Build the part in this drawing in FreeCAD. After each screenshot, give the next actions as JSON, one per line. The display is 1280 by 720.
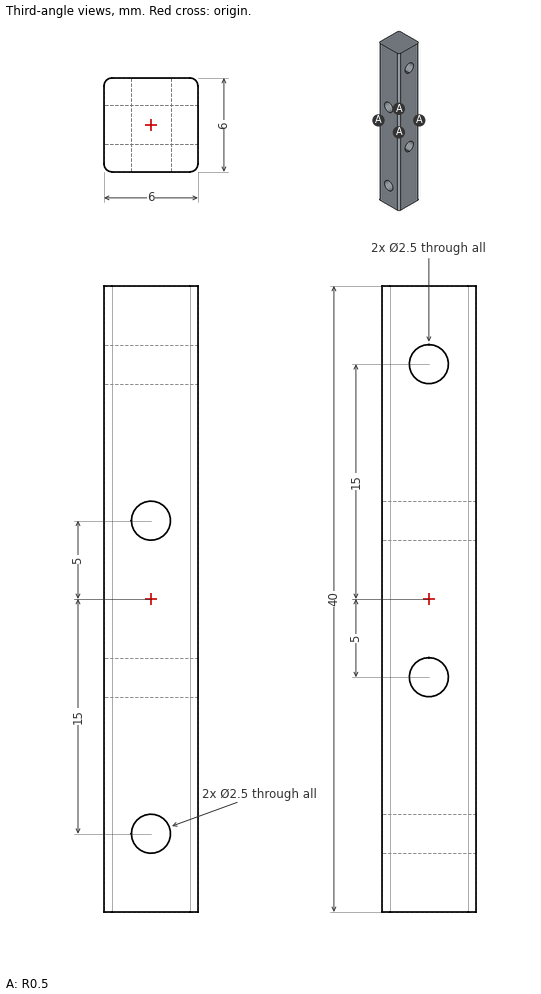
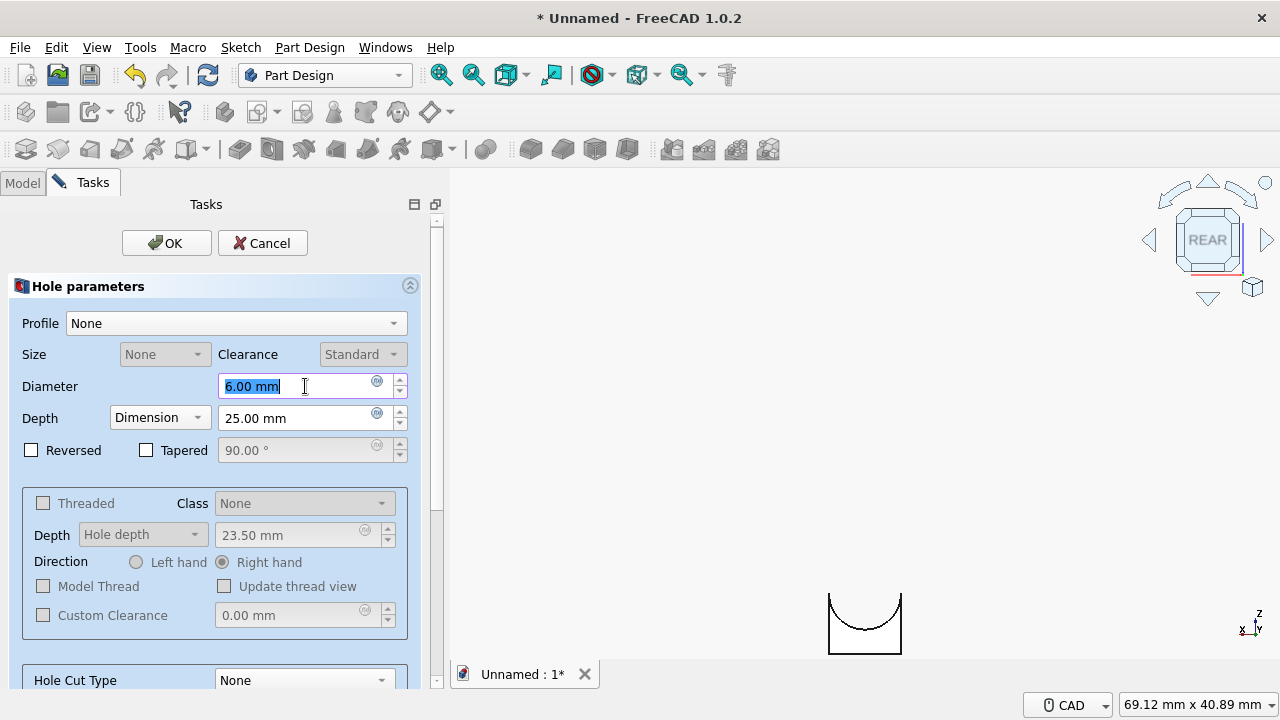
{"action": "type", "text": "2.5"}
{"action": "key", "text": "Tab"}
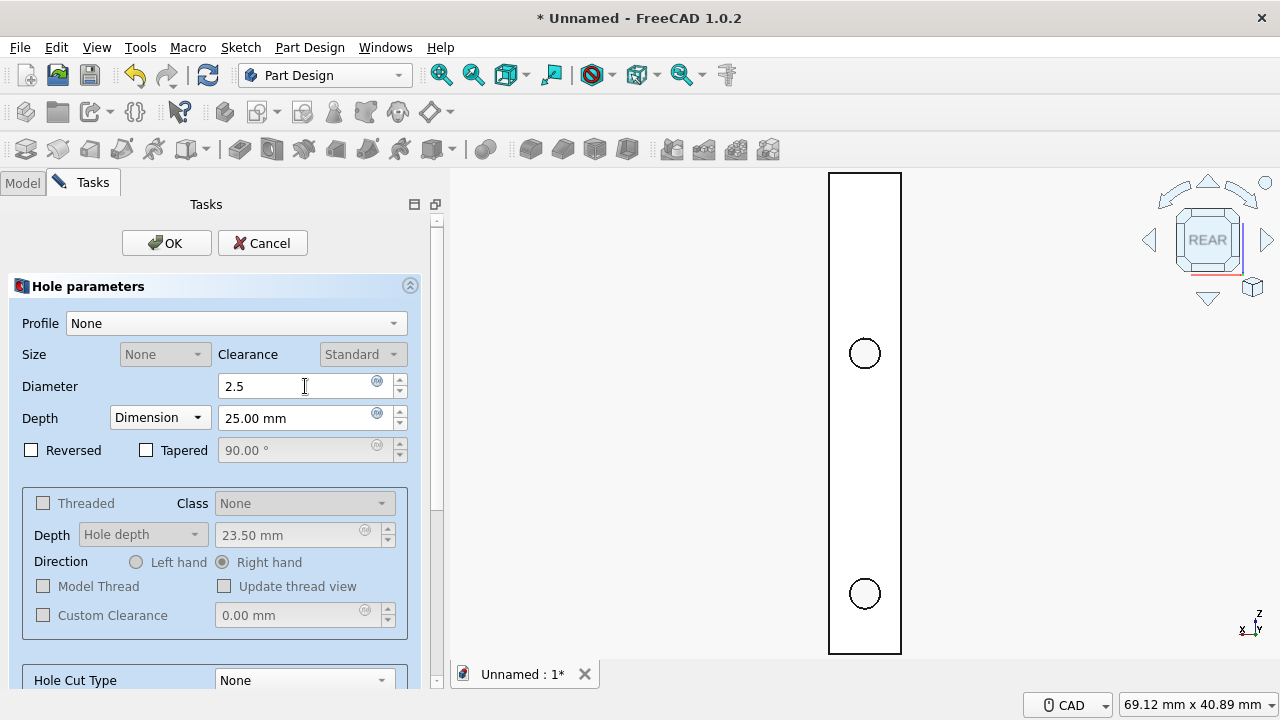
{"action": "left_click", "coordinate": [161, 418]}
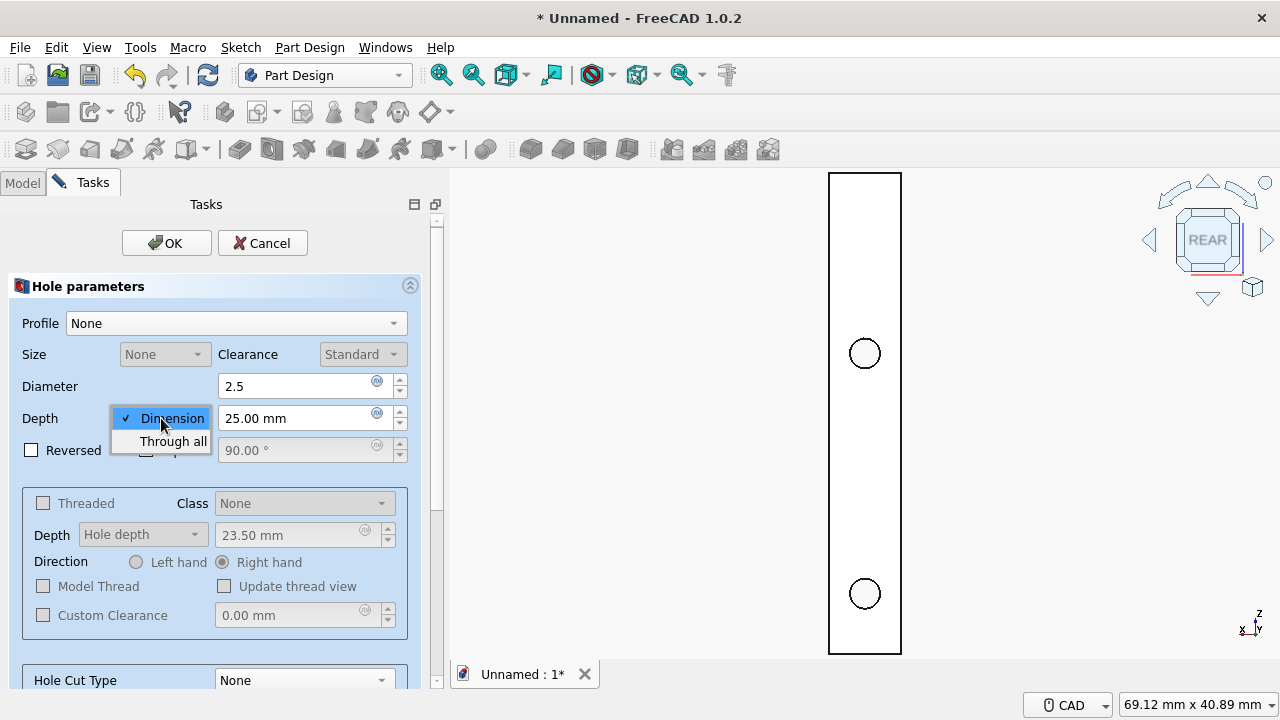
{"action": "left_click", "coordinate": [160, 442]}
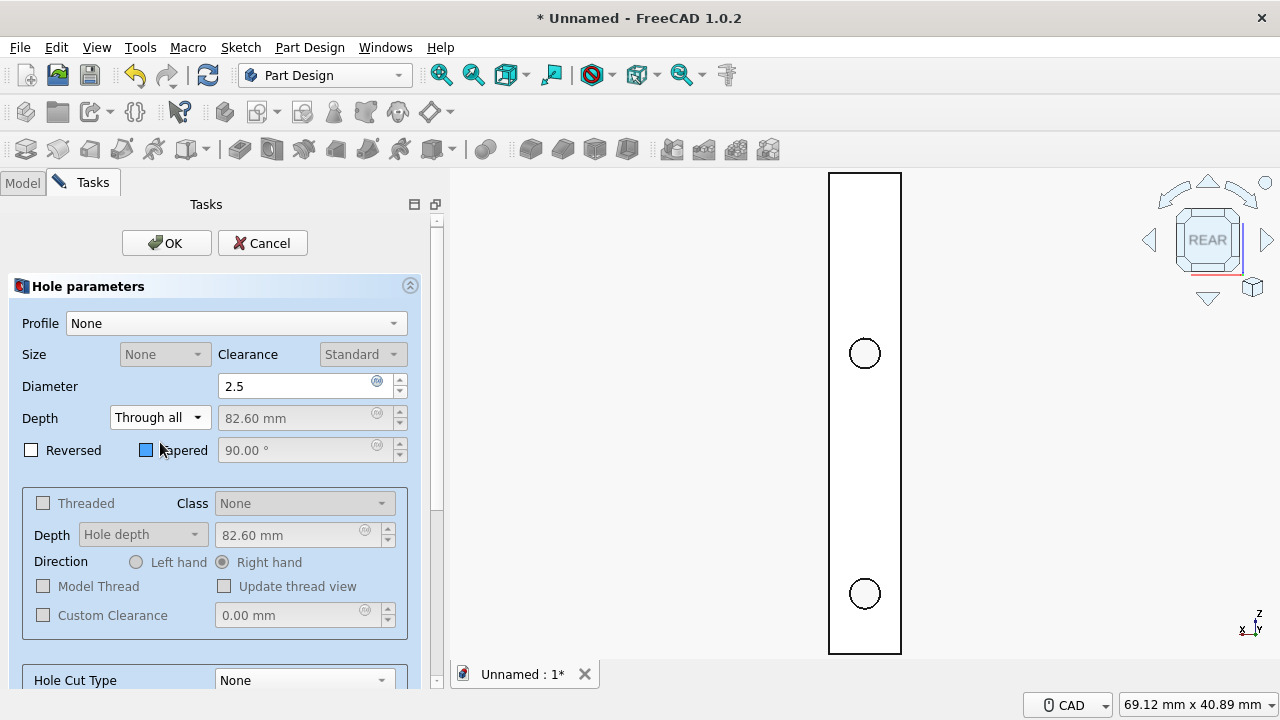
{"action": "left_click", "coordinate": [167, 243]}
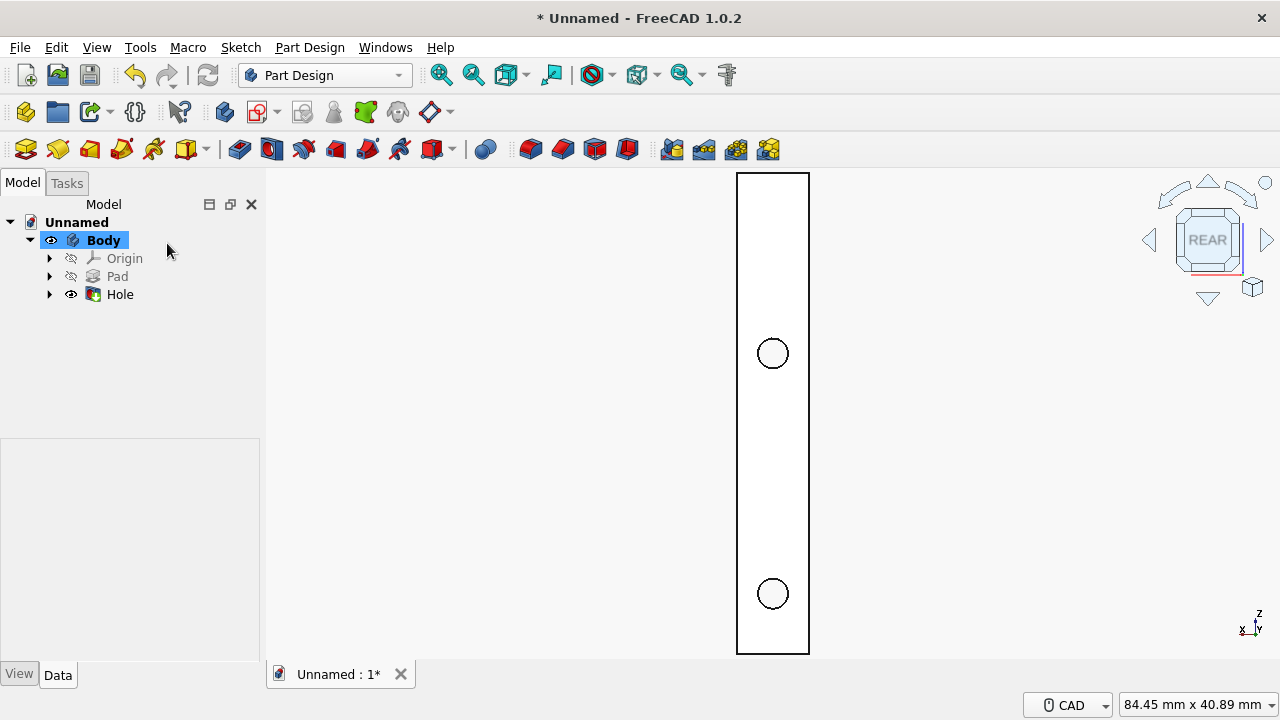
{"action": "key", "text": "0"}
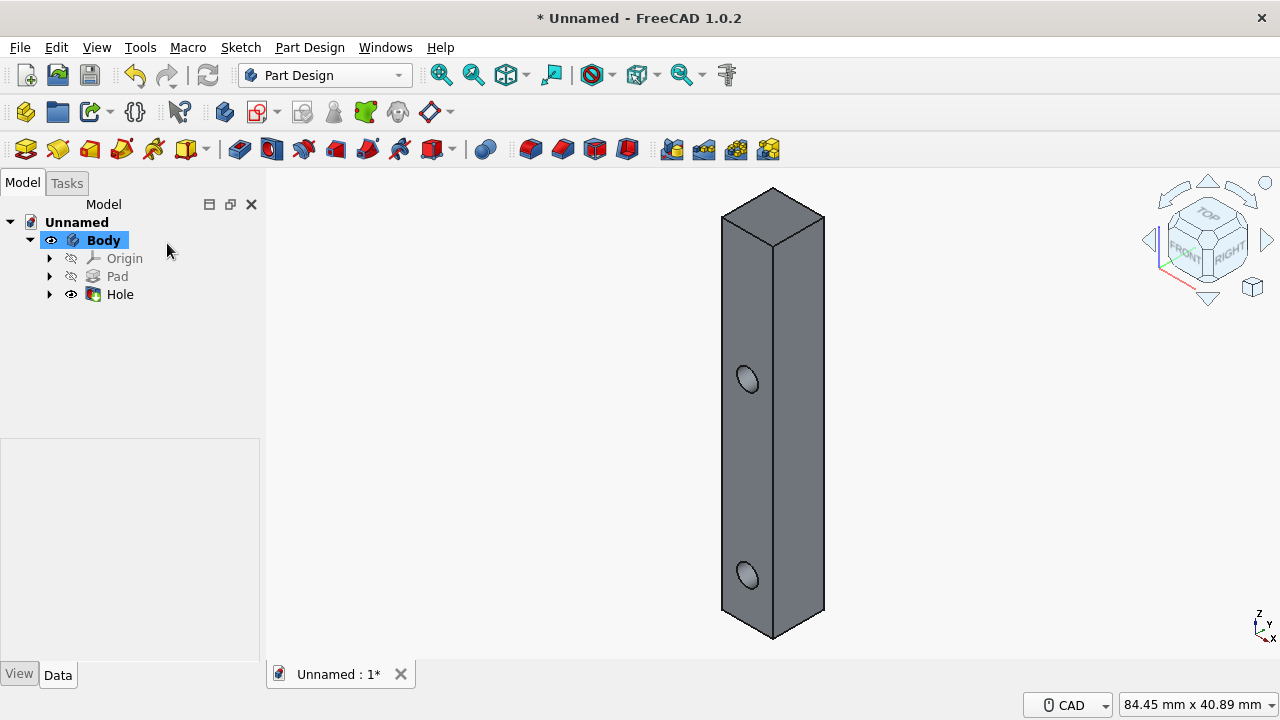
{"action": "left_click", "coordinate": [798, 315]}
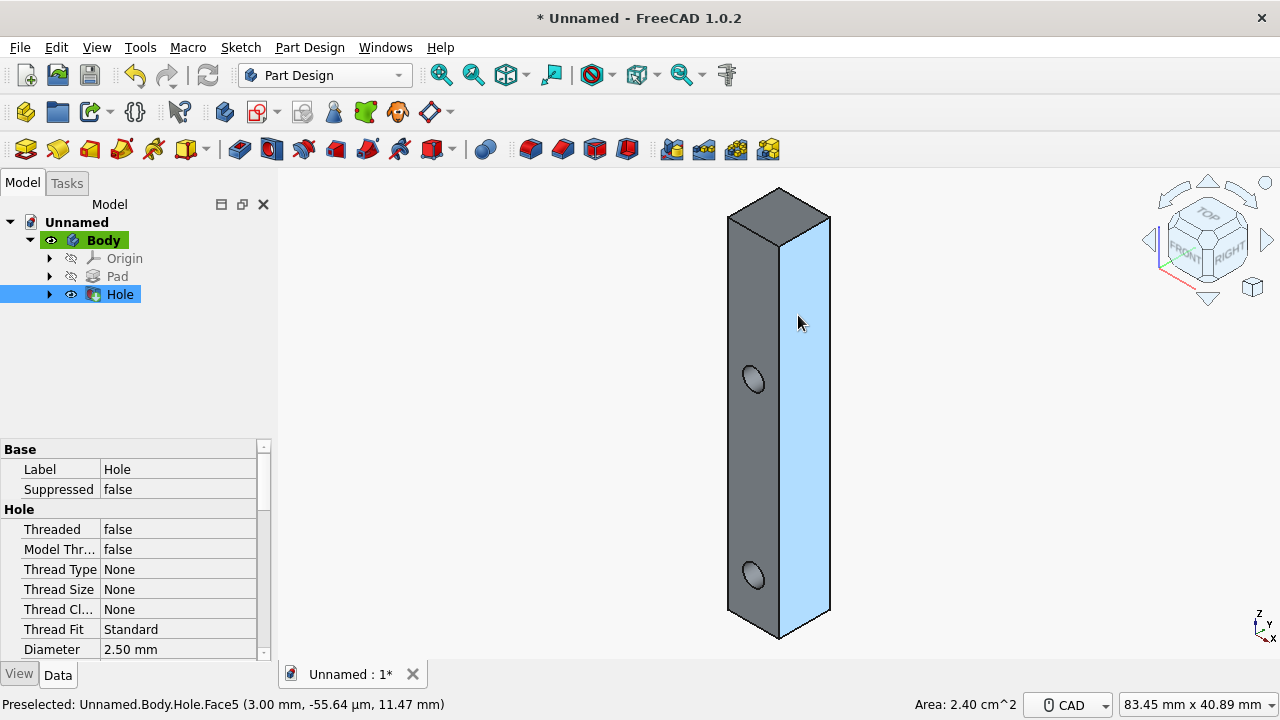
{"action": "left_click", "coordinate": [258, 112]}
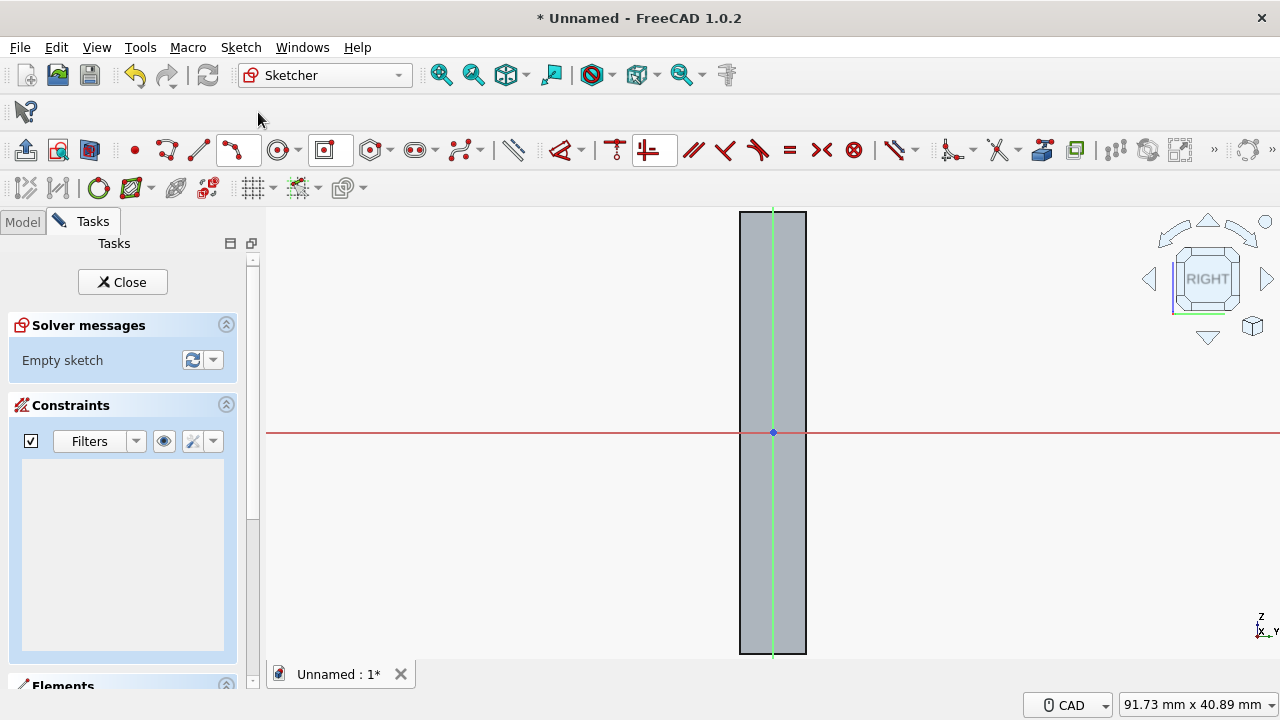
{"action": "scroll", "coordinate": [395, 631], "scroll_direction": "down", "scroll_amount": 1}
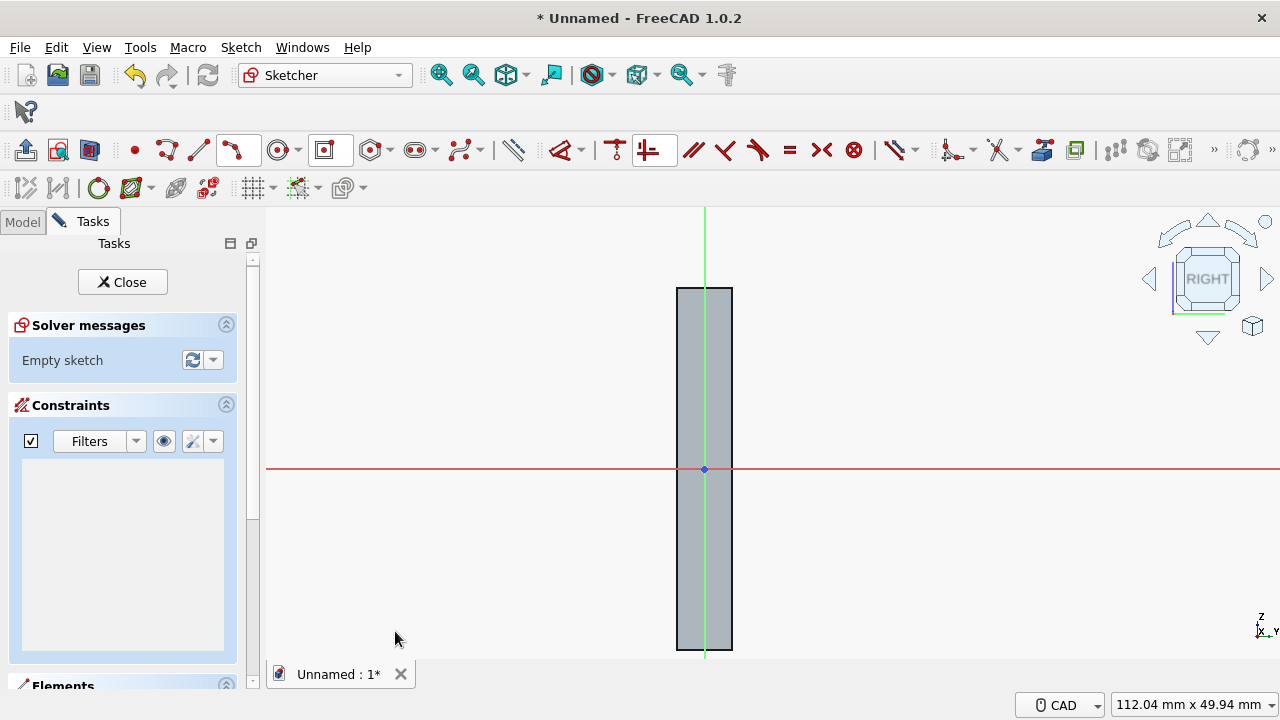
{"action": "scroll", "coordinate": [705, 405], "scroll_direction": "up", "scroll_amount": 2}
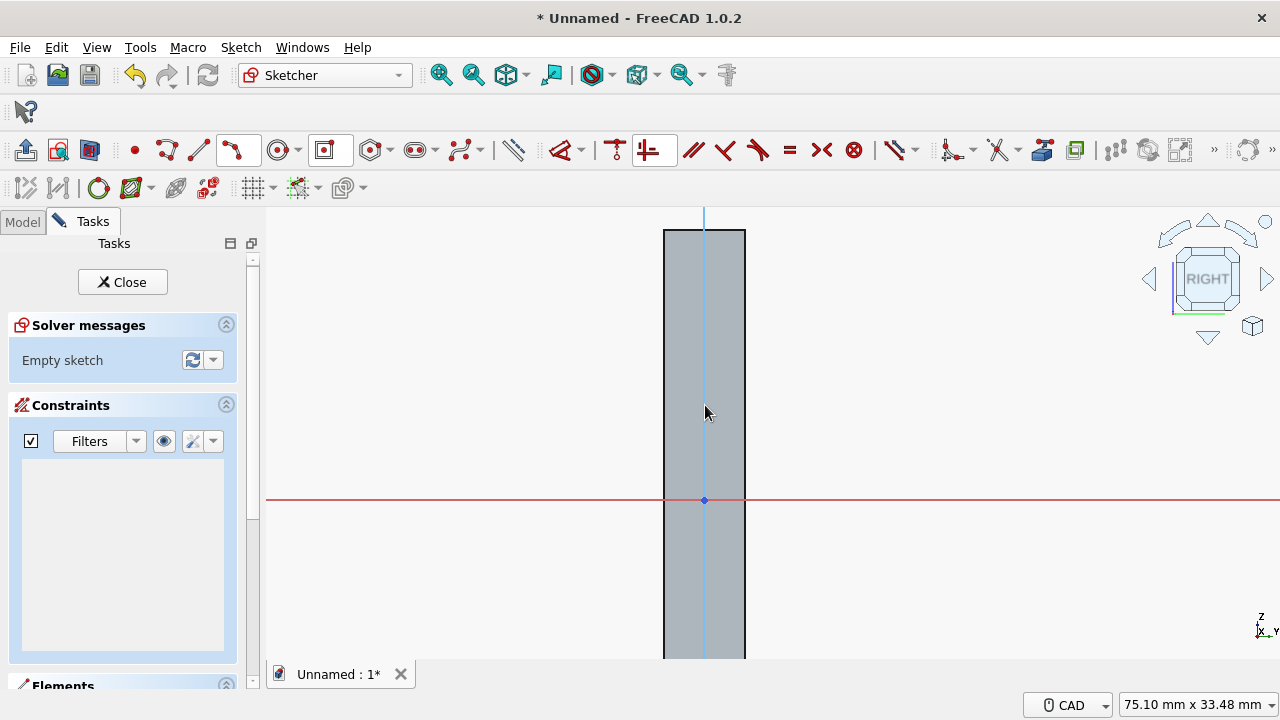
{"action": "left_click", "coordinate": [278, 150]}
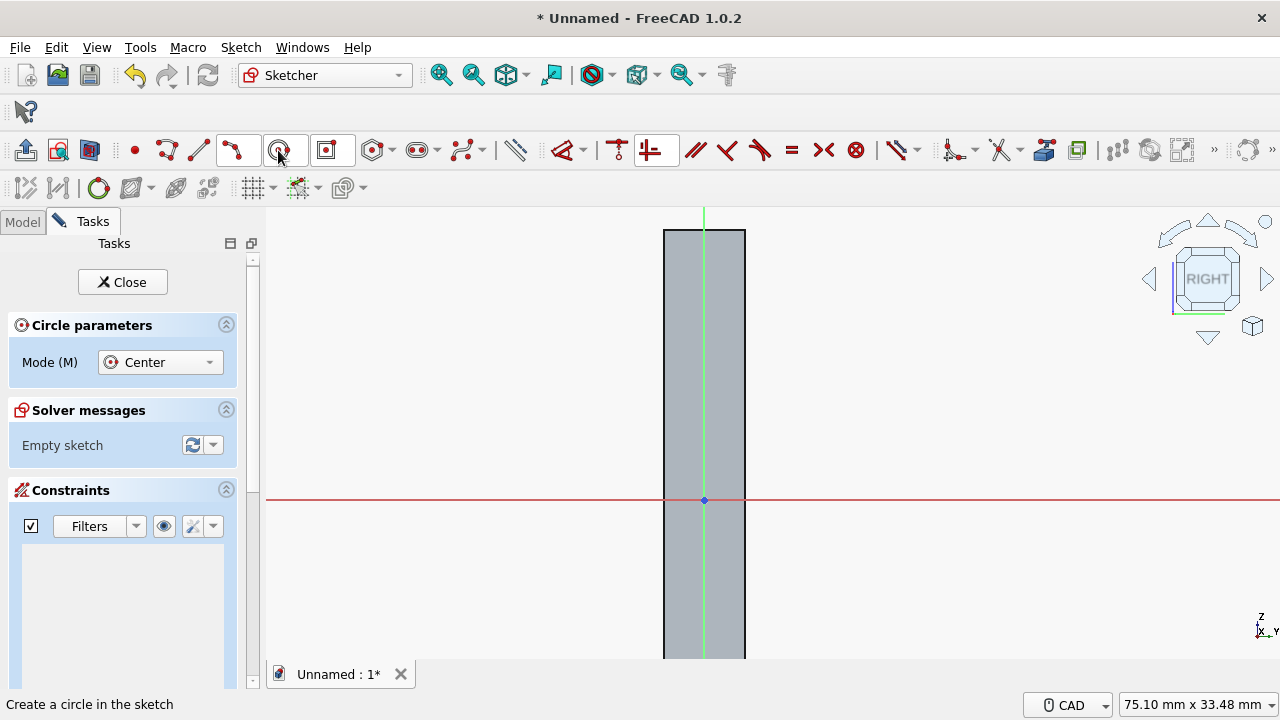
{"action": "scroll", "coordinate": [704, 298], "scroll_direction": "up", "scroll_amount": 2}